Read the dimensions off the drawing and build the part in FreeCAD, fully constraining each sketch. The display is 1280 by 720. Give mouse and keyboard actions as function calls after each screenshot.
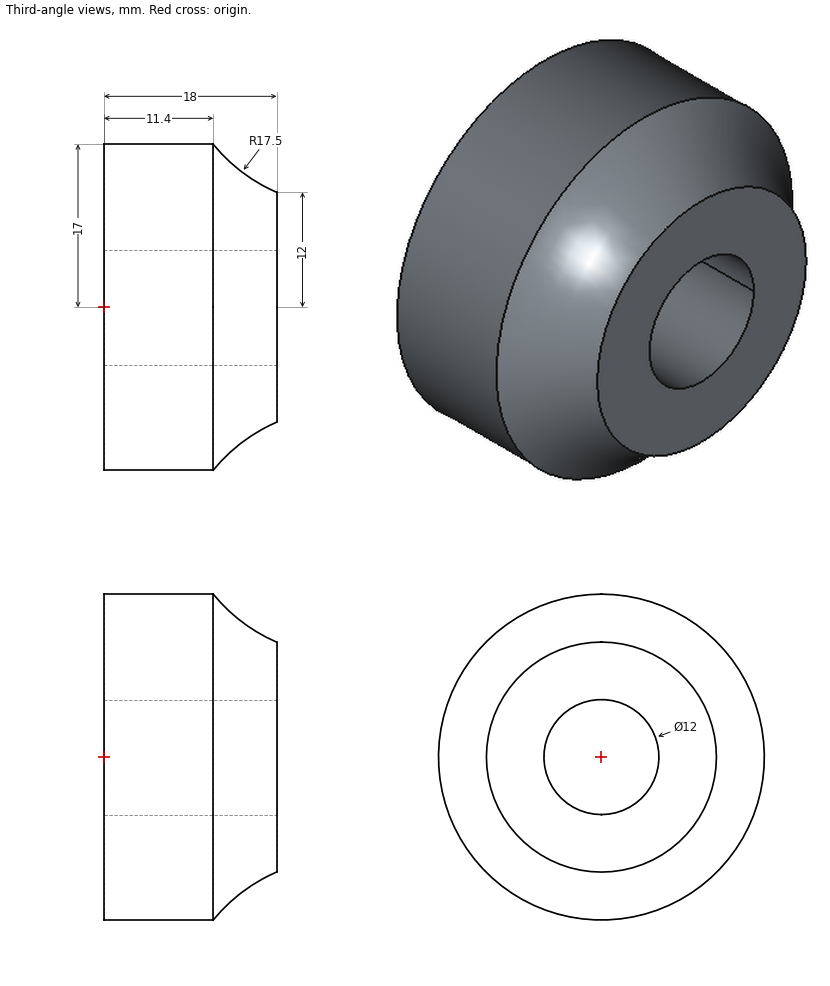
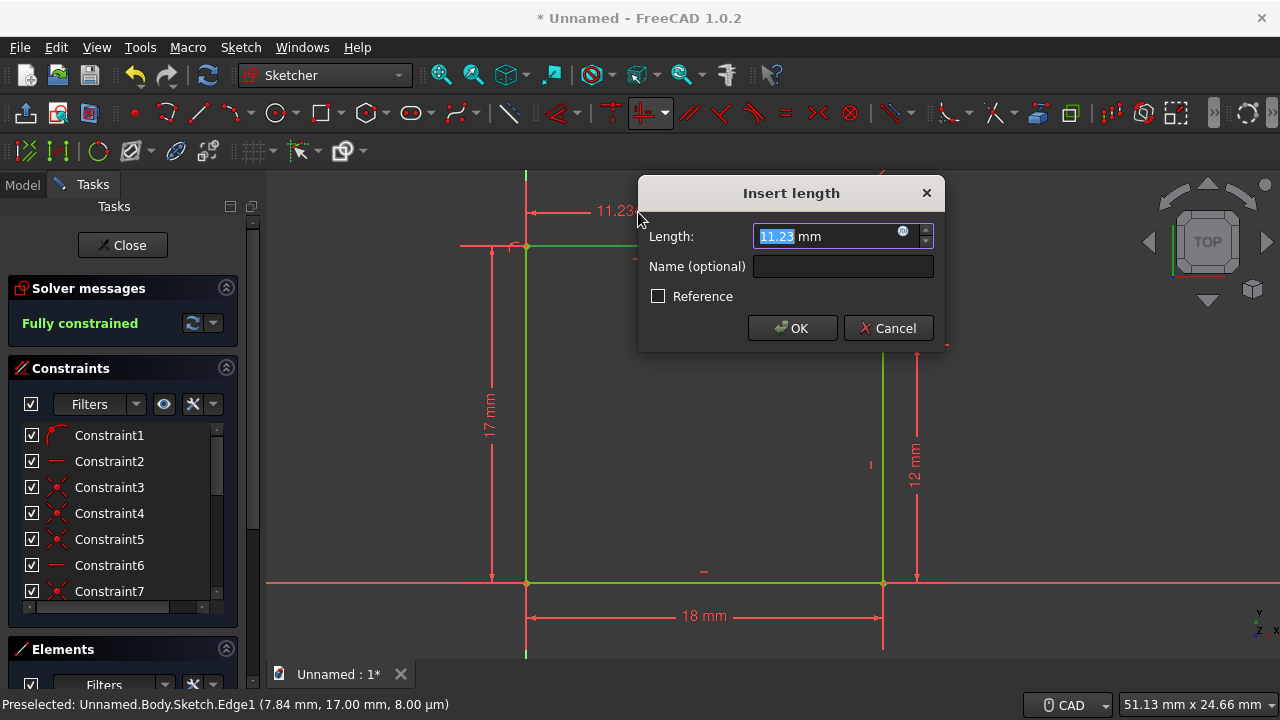
text(11.4)
key(Return)
key(Escape)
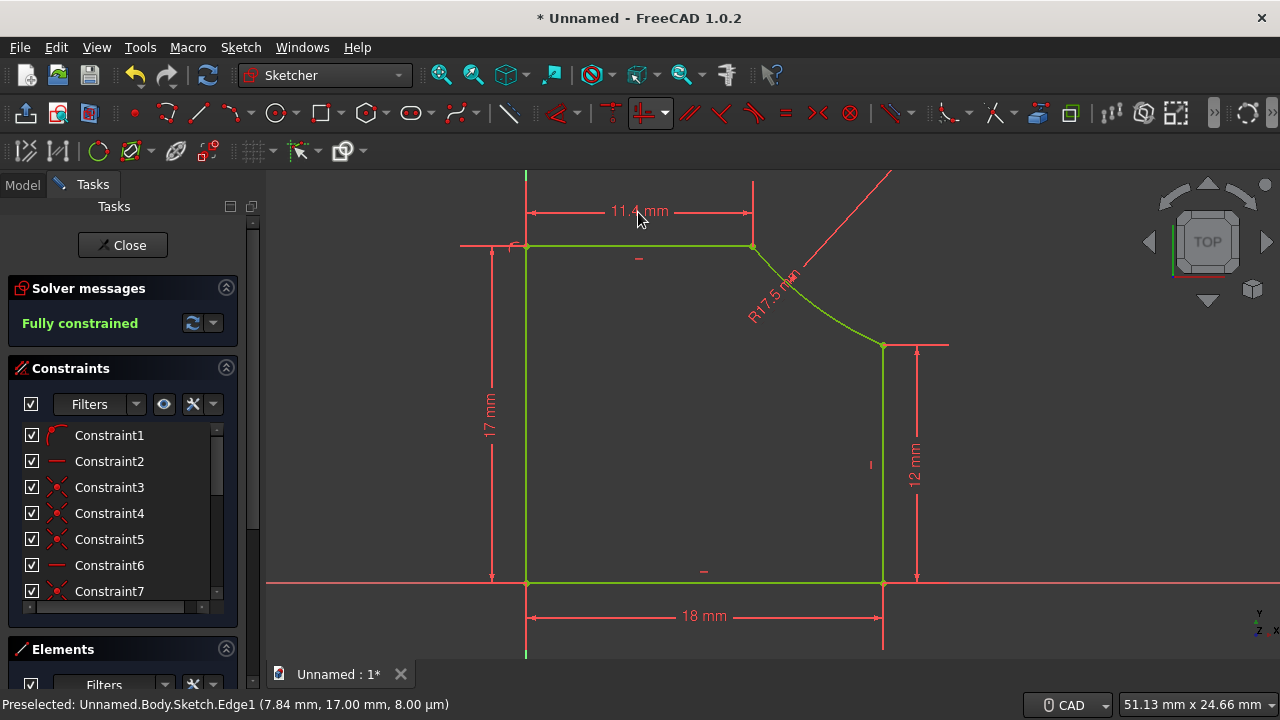
click(123, 245)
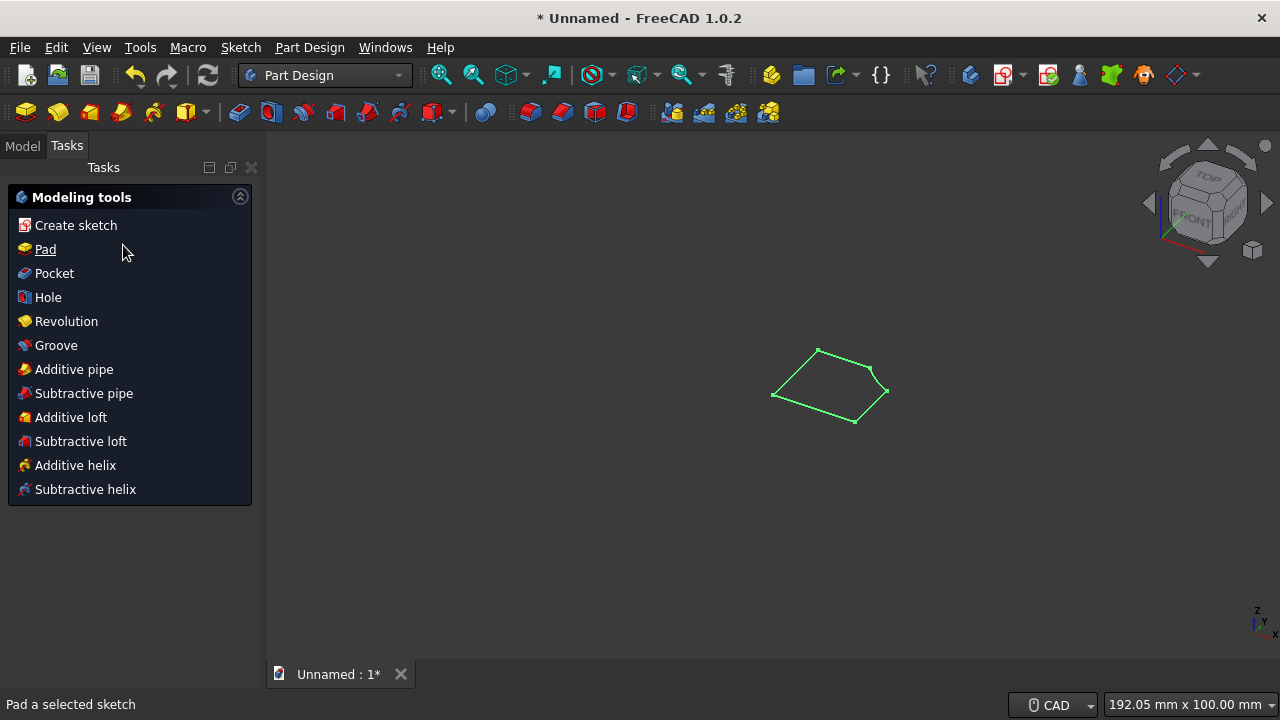
click(58, 112)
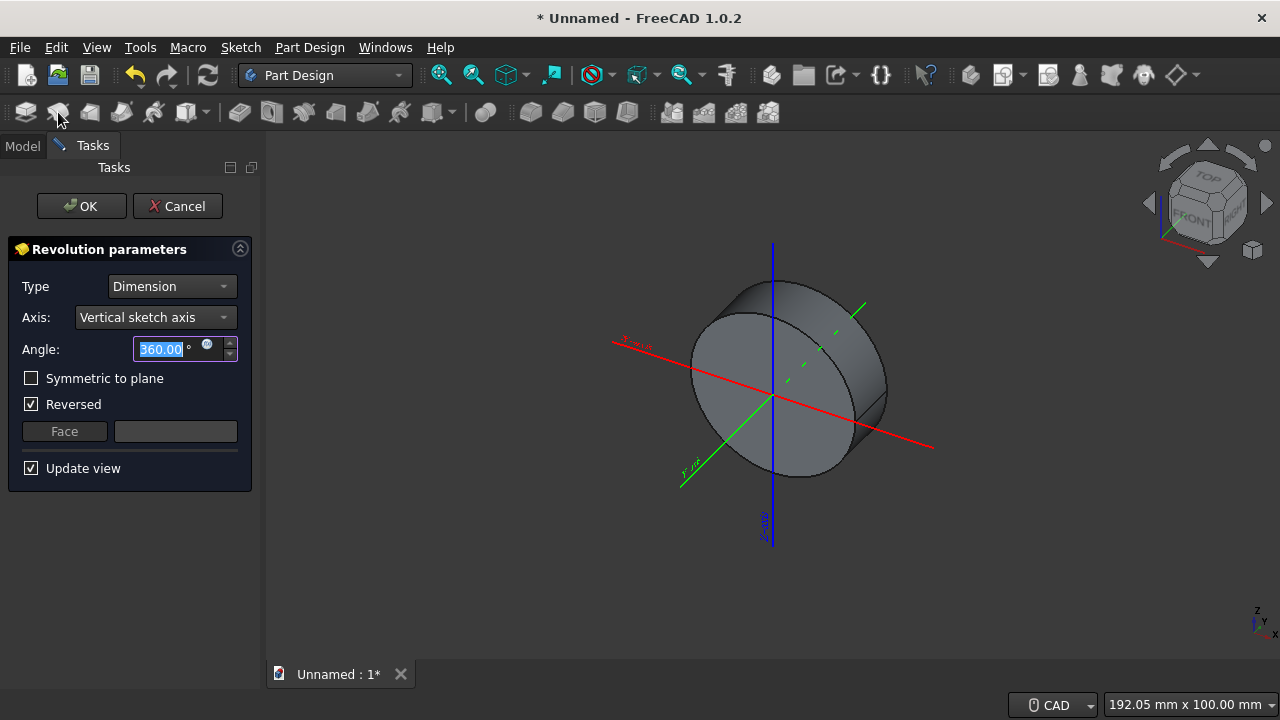
click(156, 318)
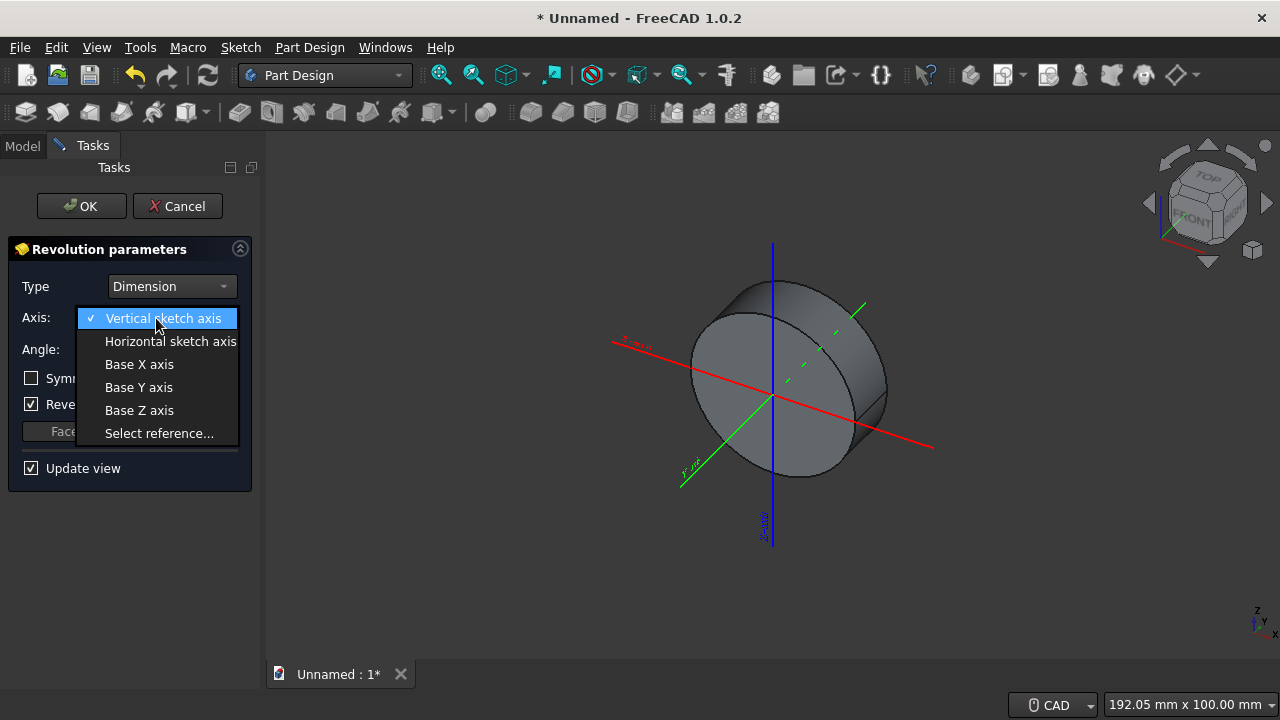
click(156, 342)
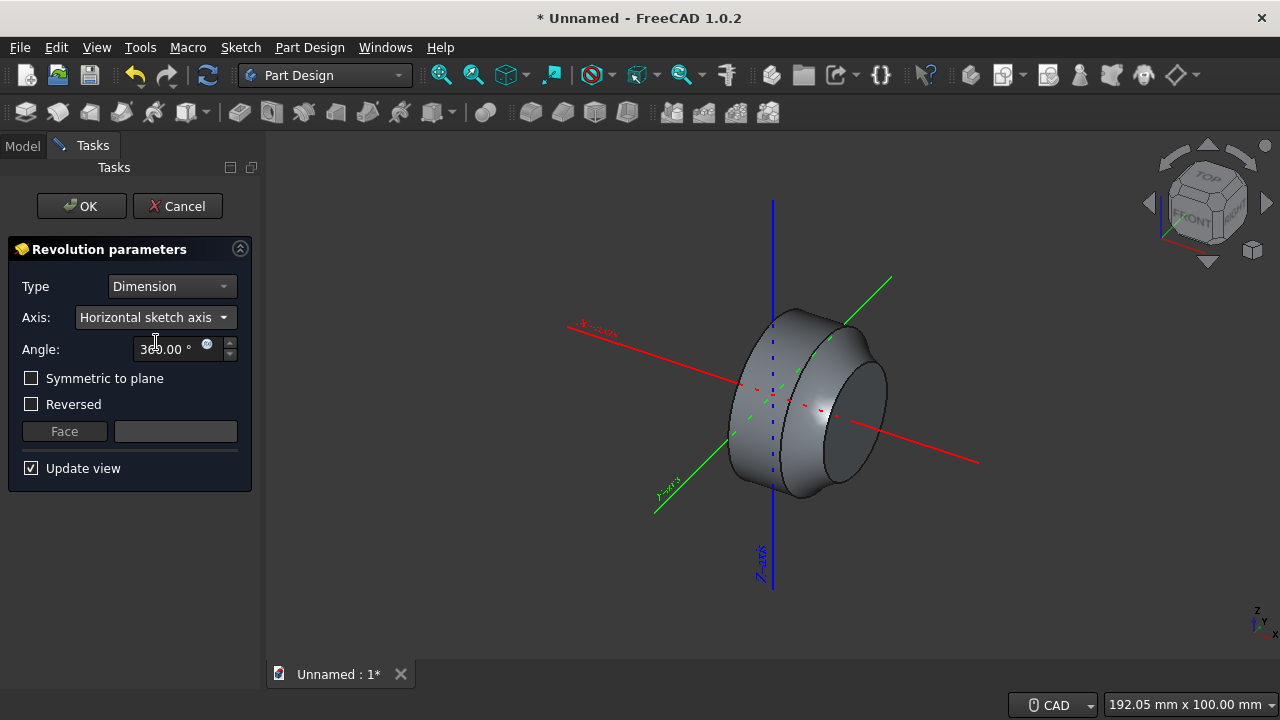
click(82, 206)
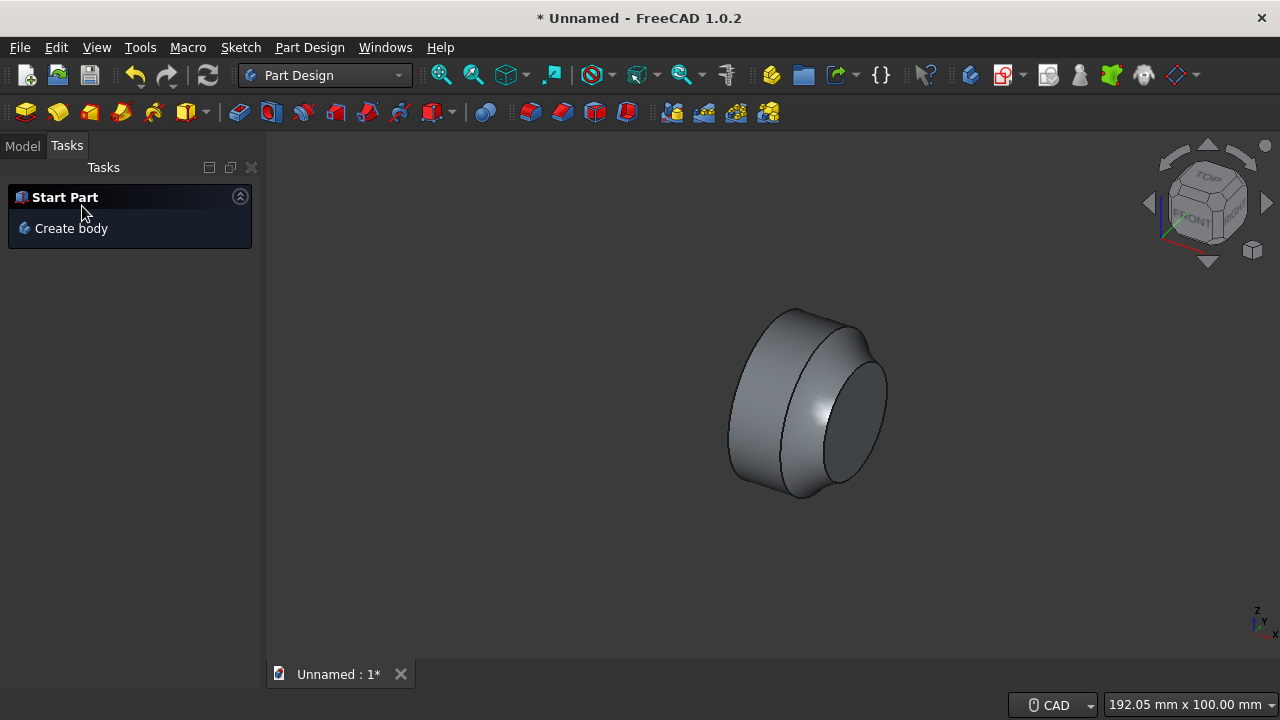
click(855, 421)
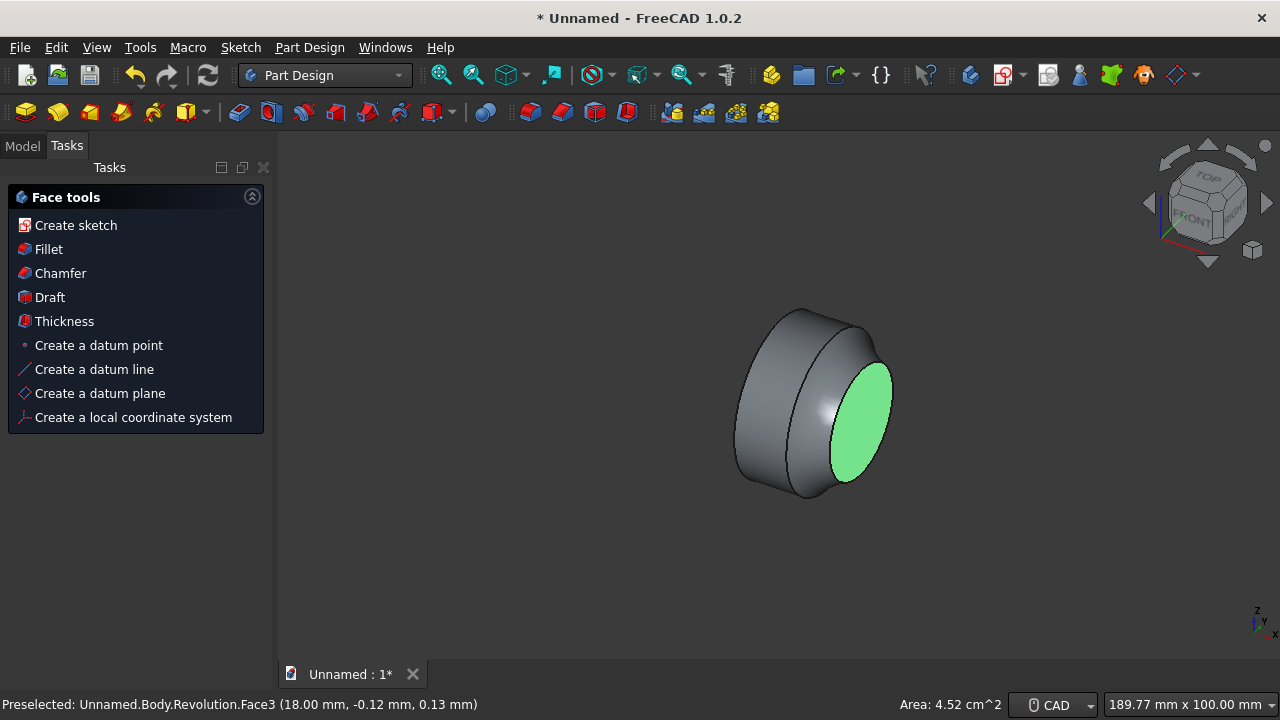
click(1004, 76)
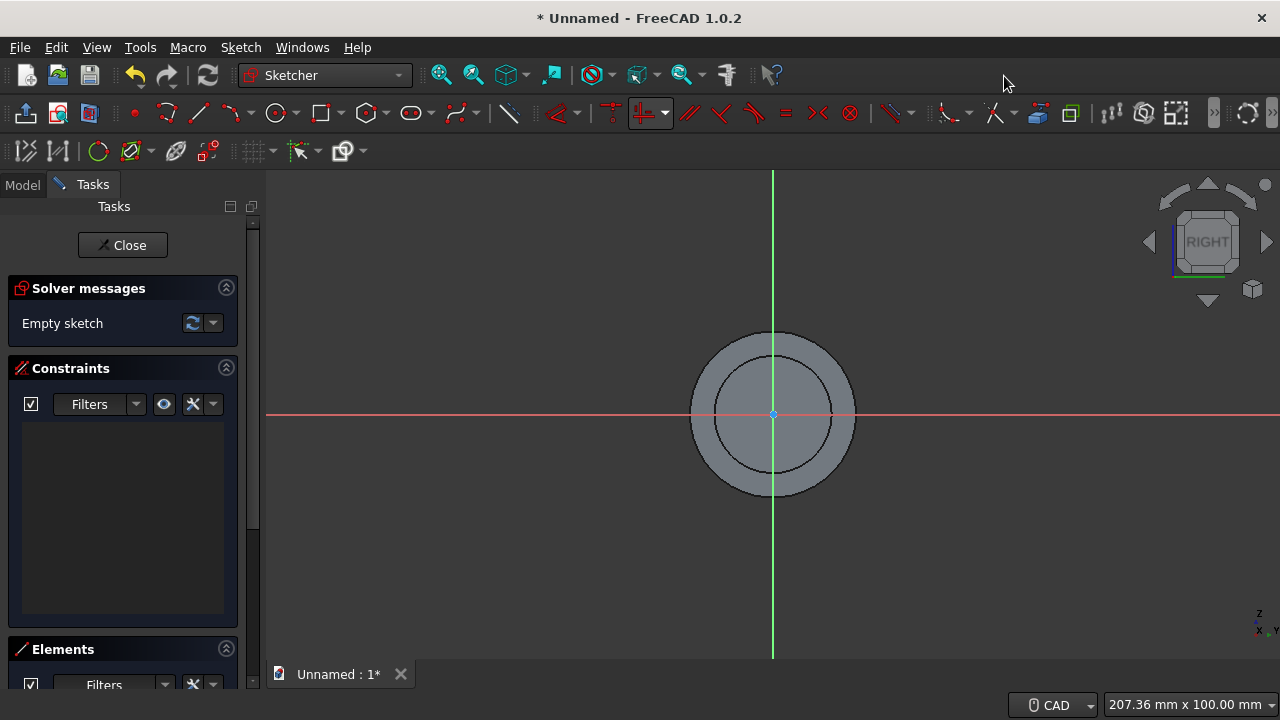
scroll(790, 414, up, 8)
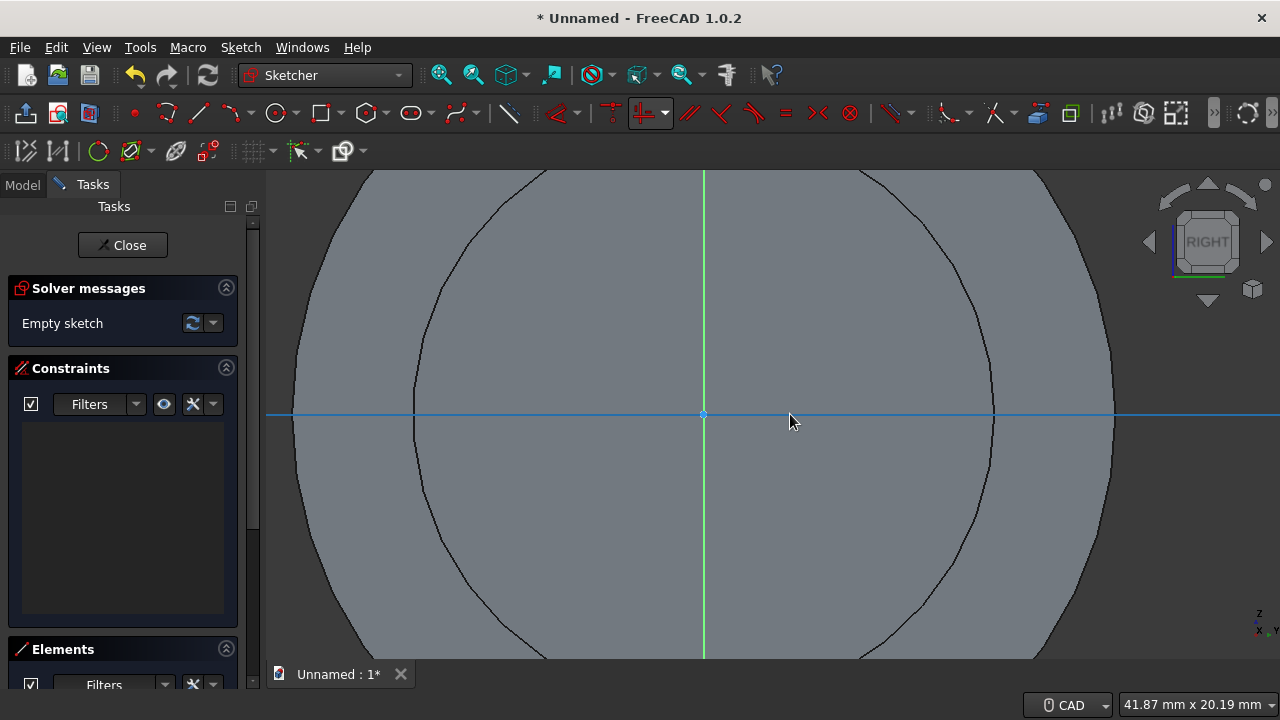
click(276, 114)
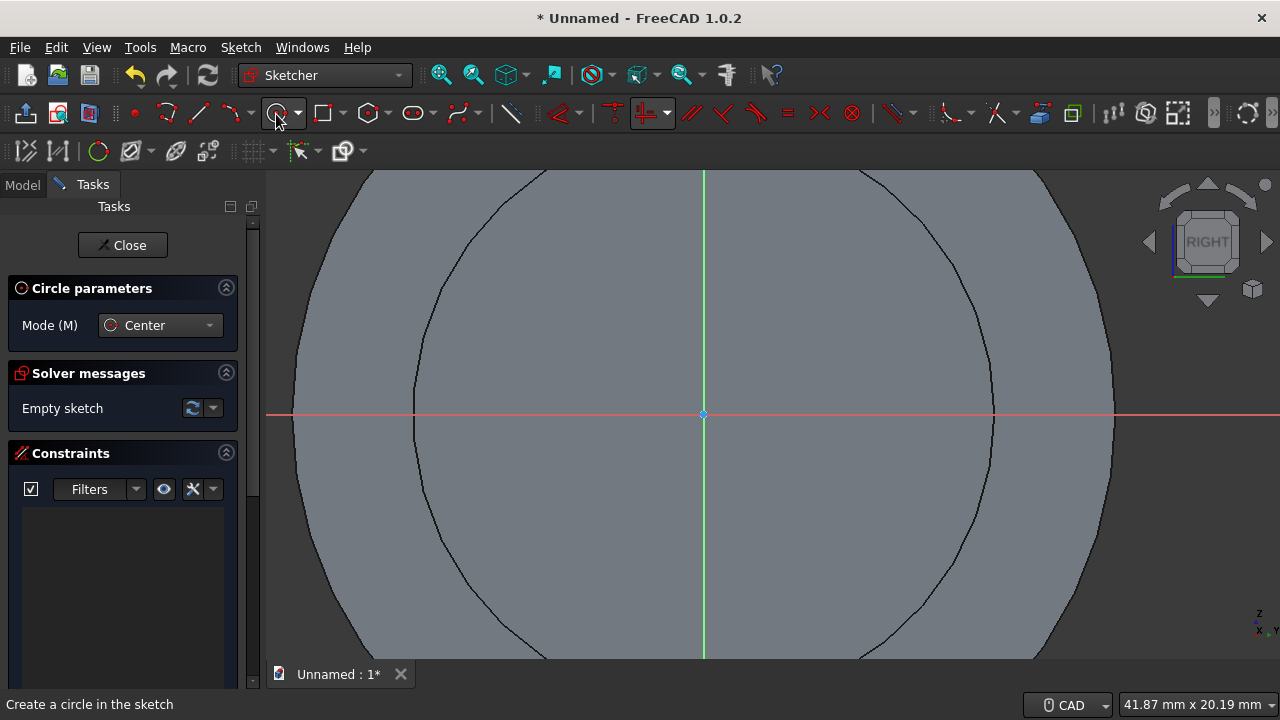
click(704, 414)
click(807, 312)
key(Escape)